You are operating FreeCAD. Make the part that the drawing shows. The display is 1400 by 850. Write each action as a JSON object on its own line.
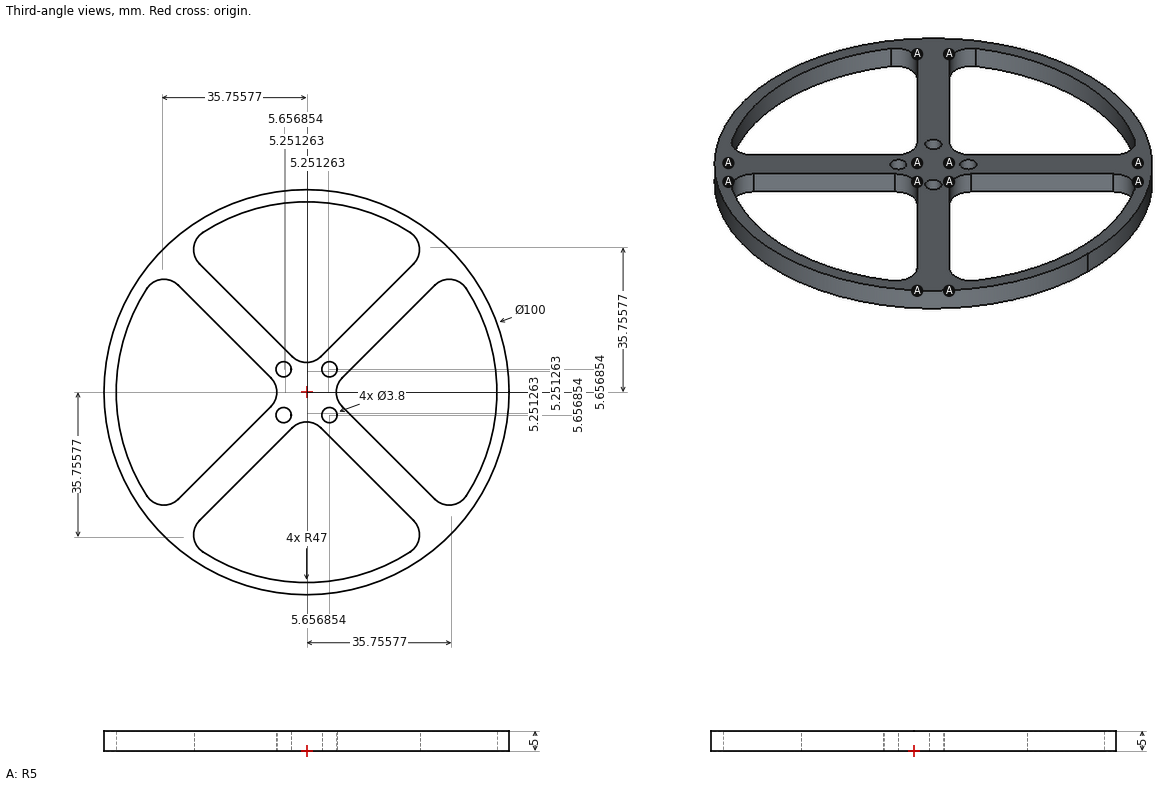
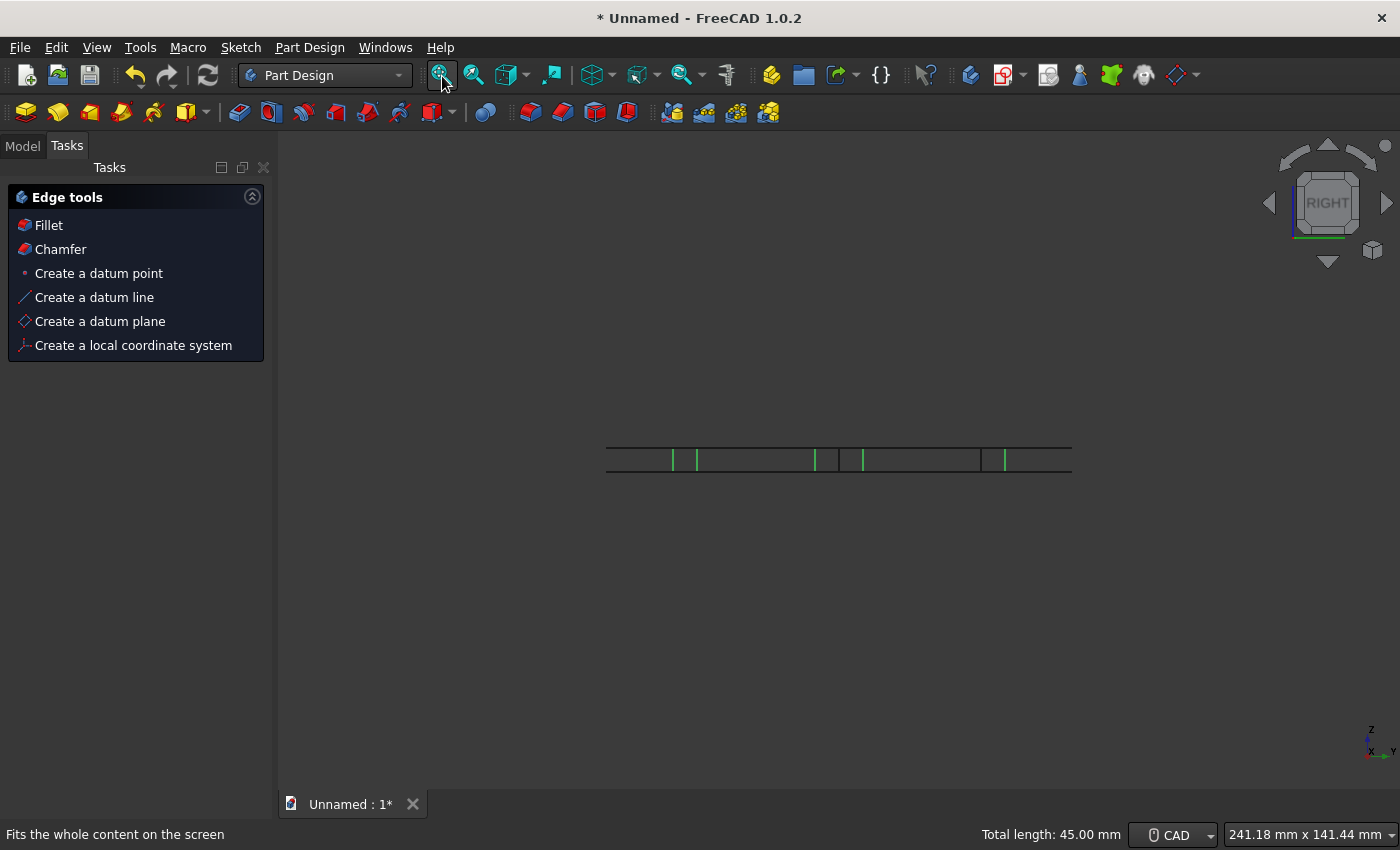
{"action": "left_click", "coordinate": [981, 459], "text": "ctrl"}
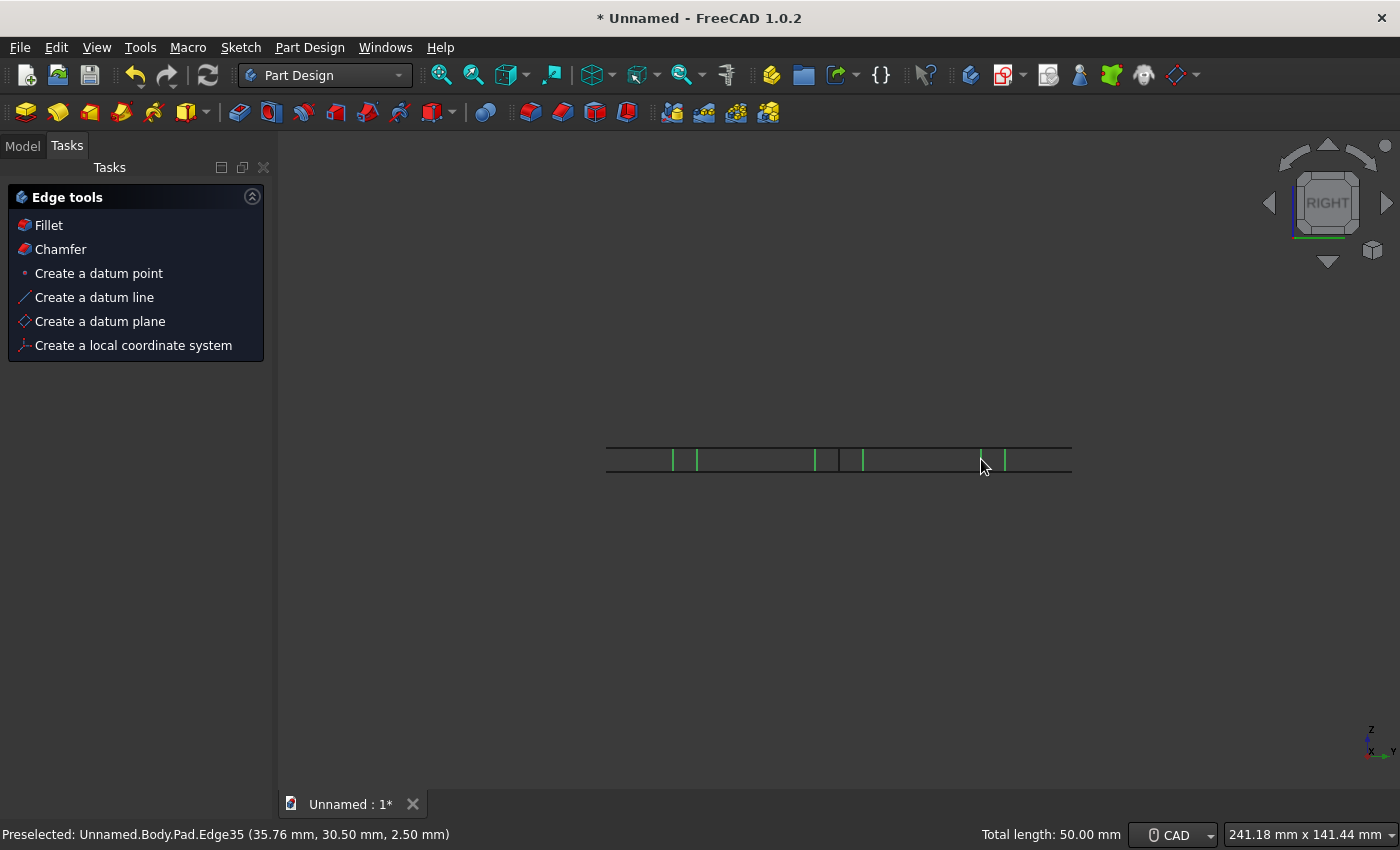
{"action": "key", "text": "5"}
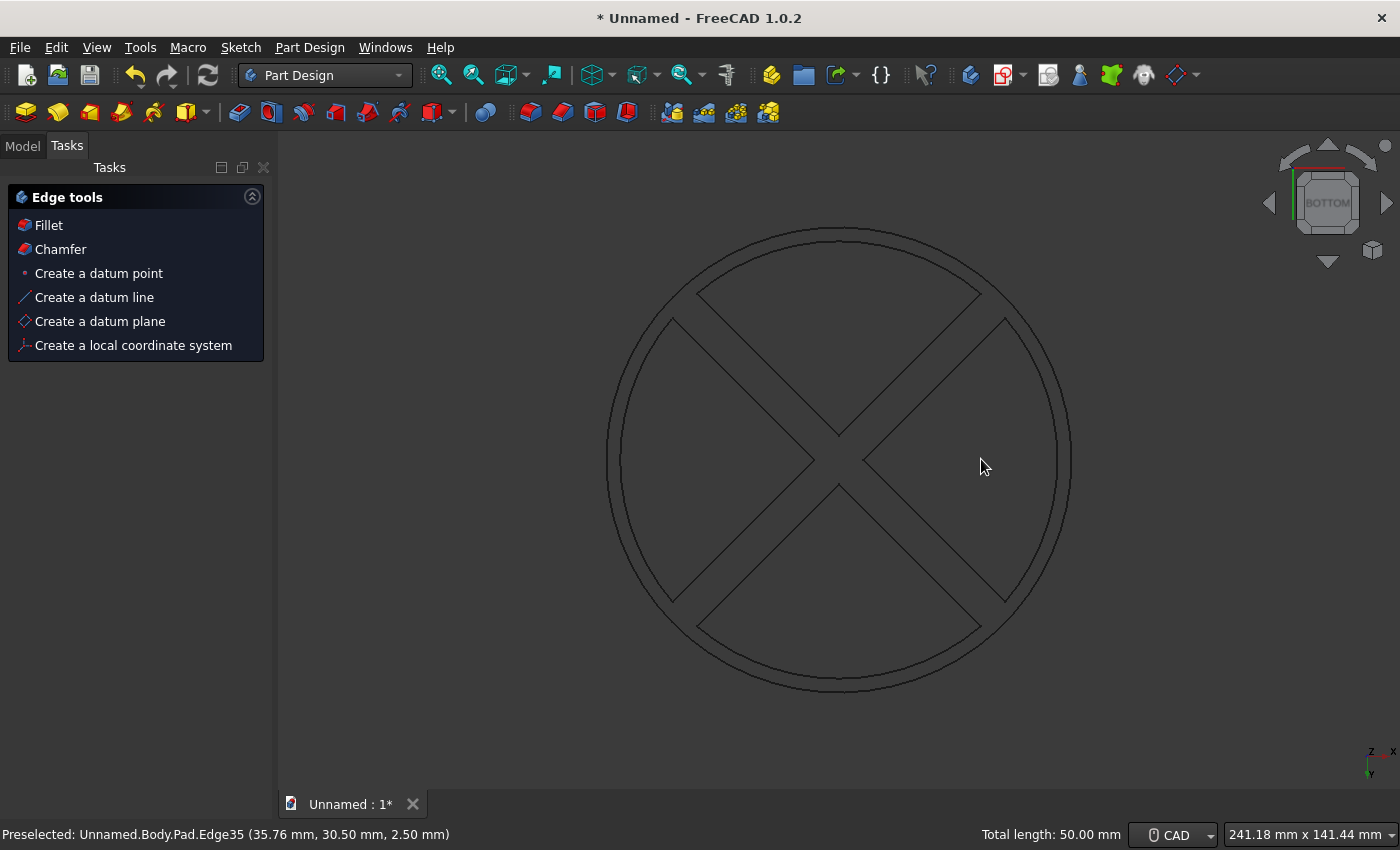
{"action": "key", "text": "4"}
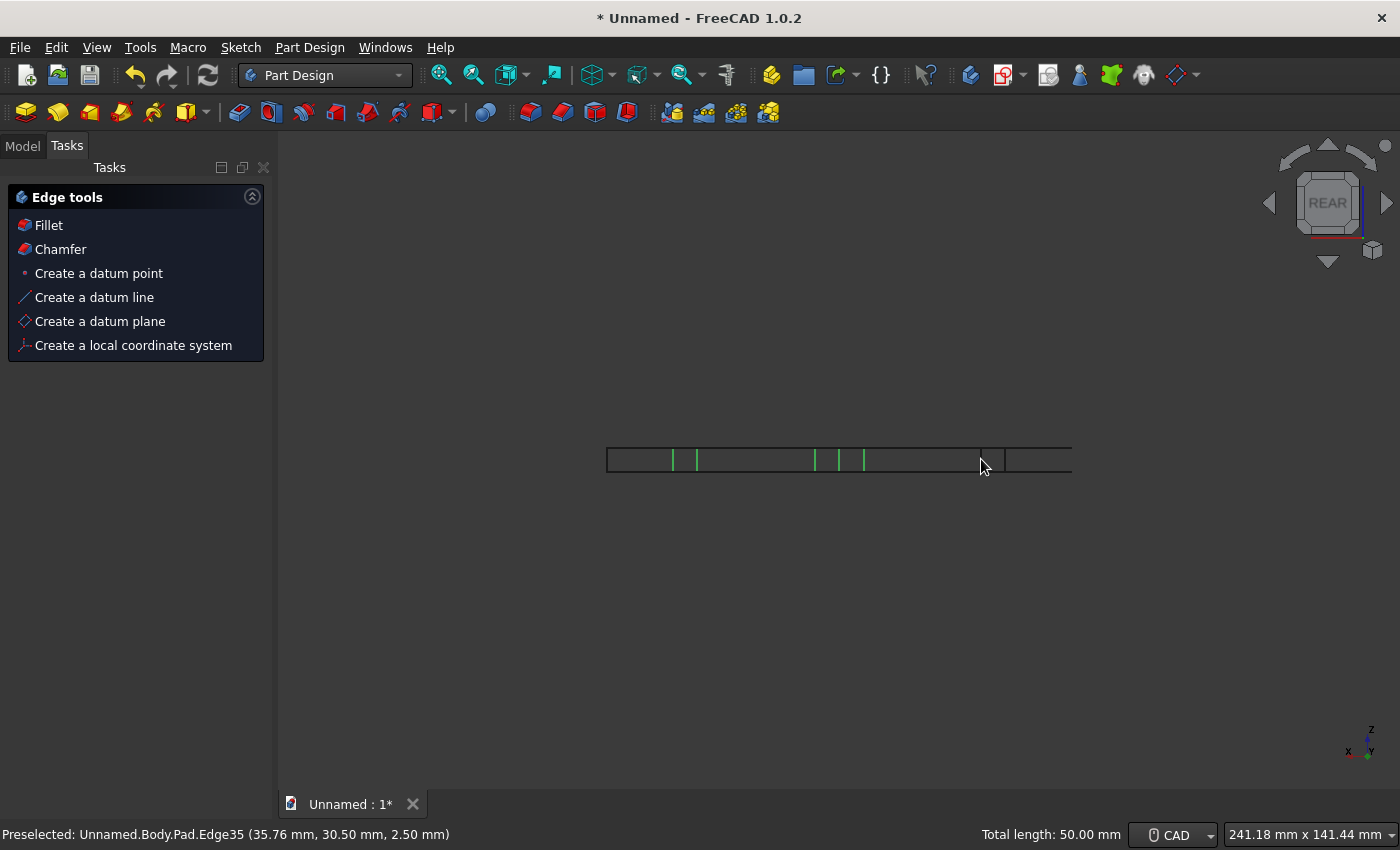
{"action": "left_click", "coordinate": [442, 76]}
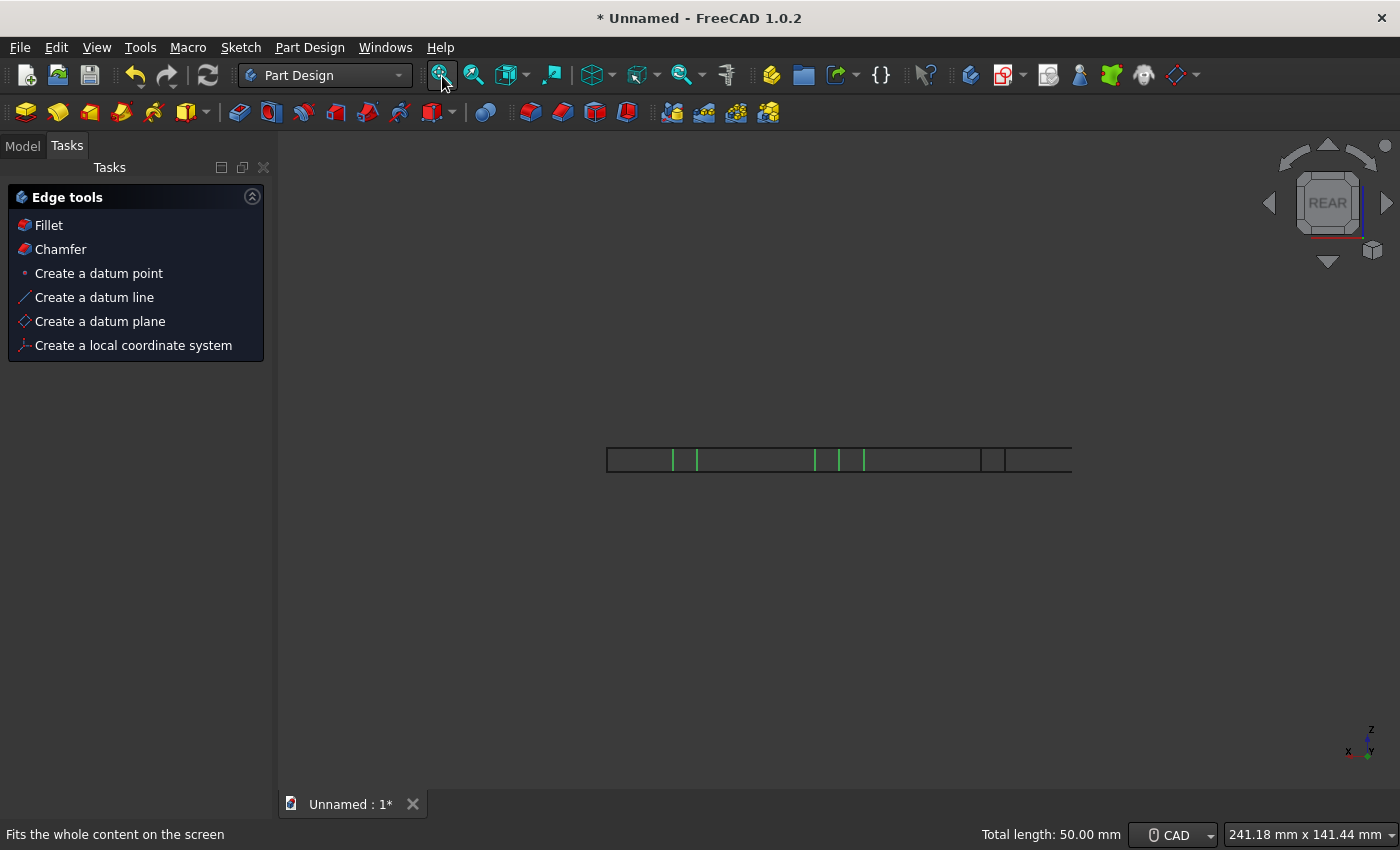
{"action": "left_click", "coordinate": [1005, 459], "text": "ctrl"}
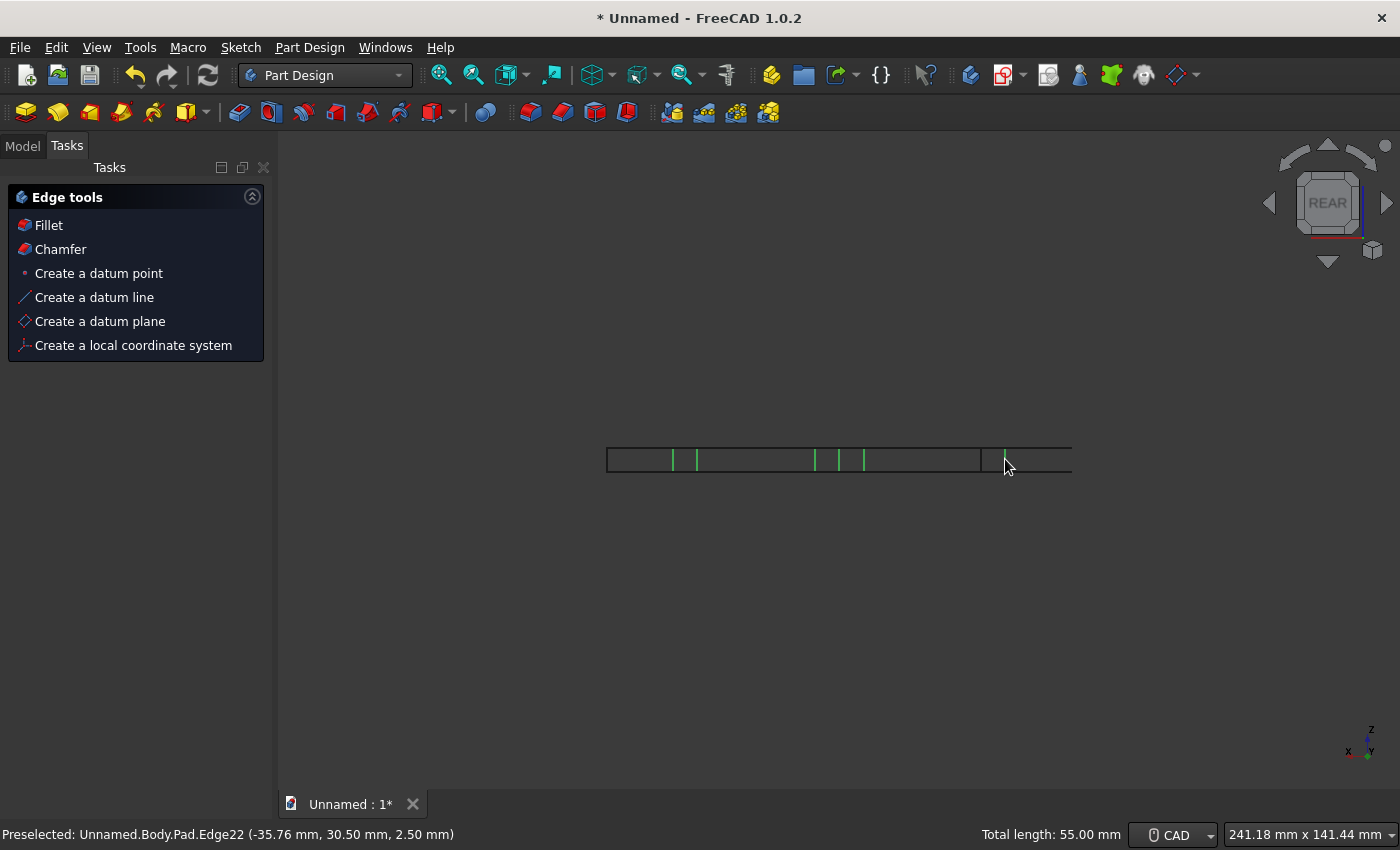
{"action": "left_click", "coordinate": [981, 459], "text": "ctrl"}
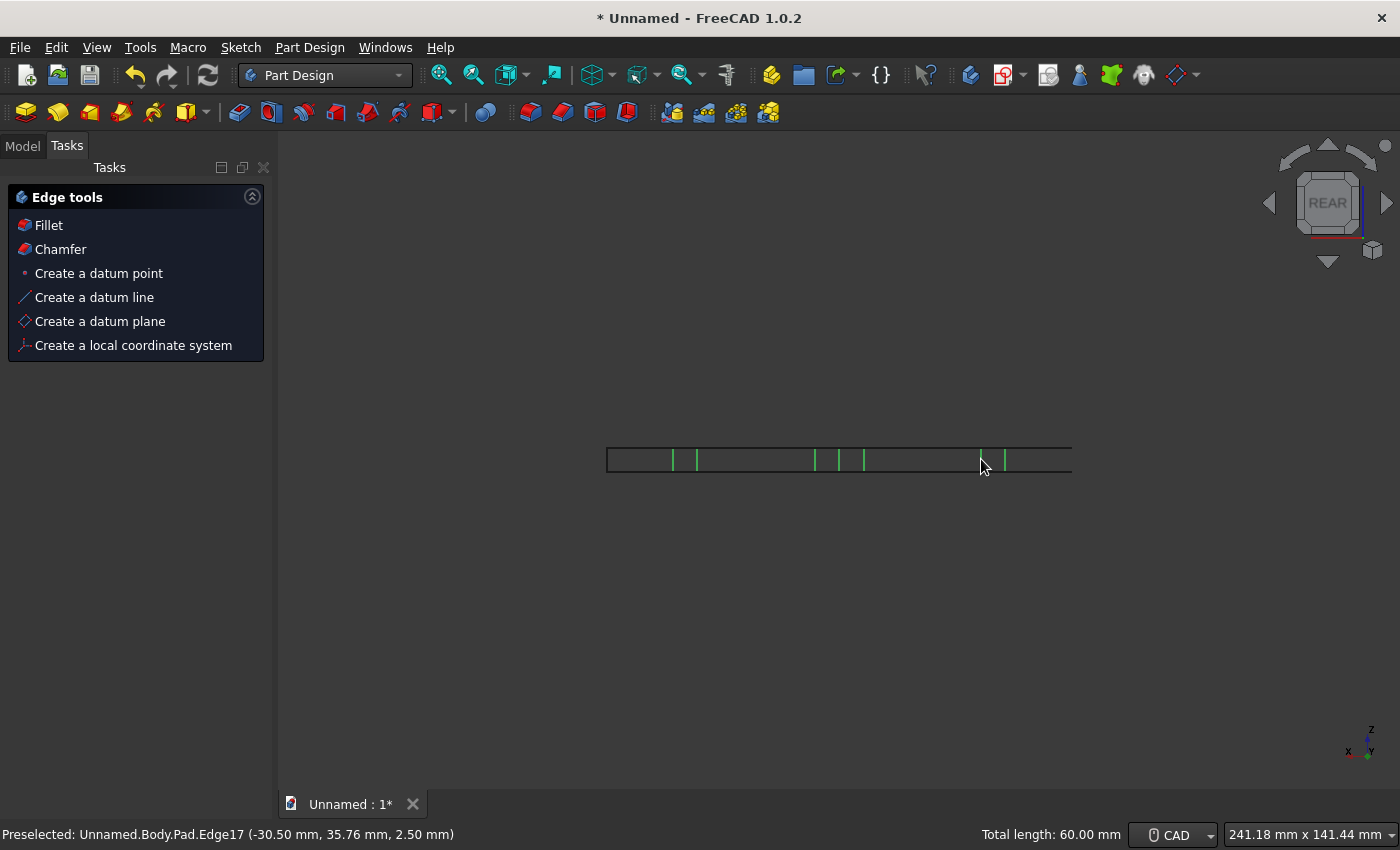
{"action": "key", "text": "v 1"}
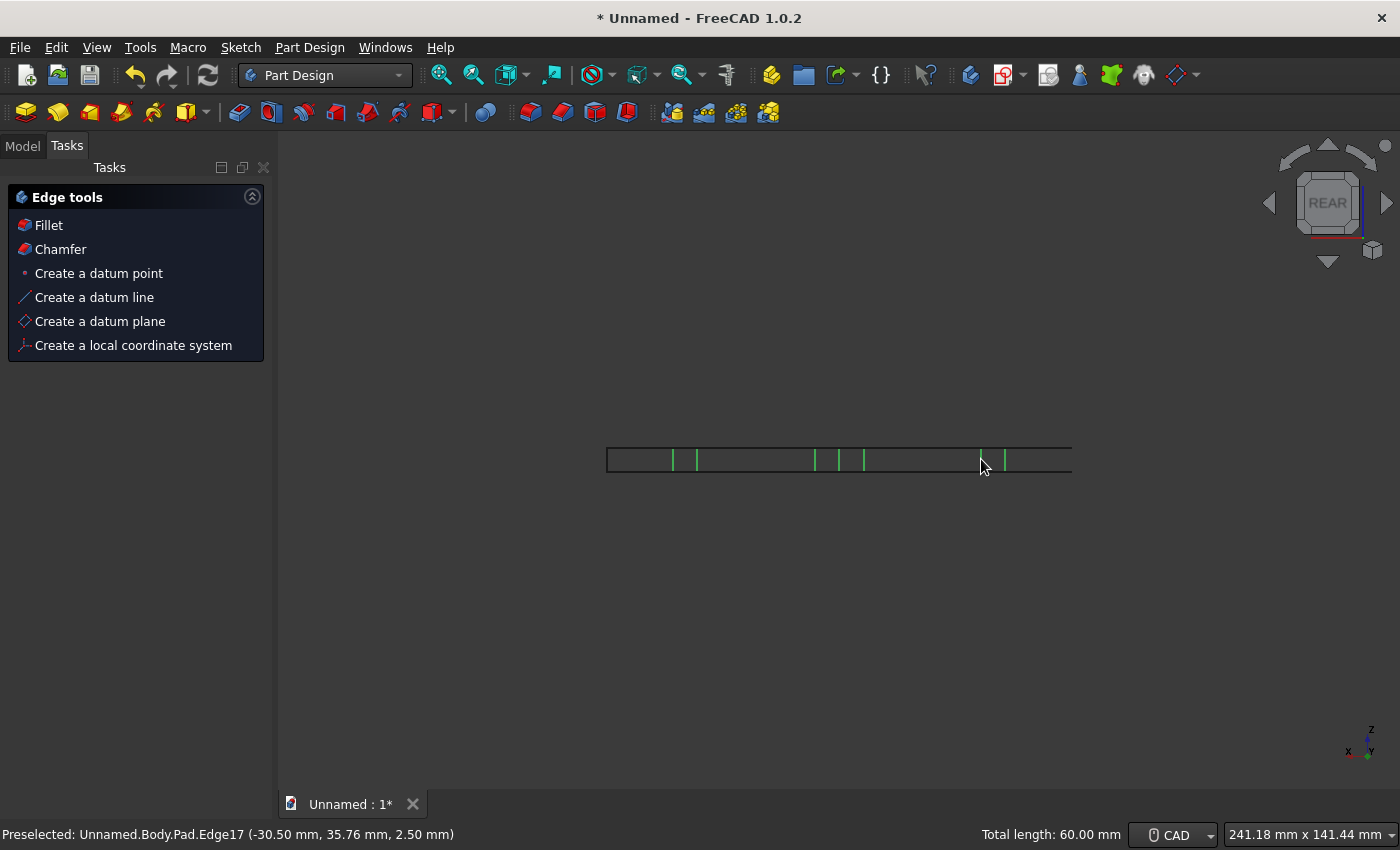
{"action": "left_click", "coordinate": [532, 112]}